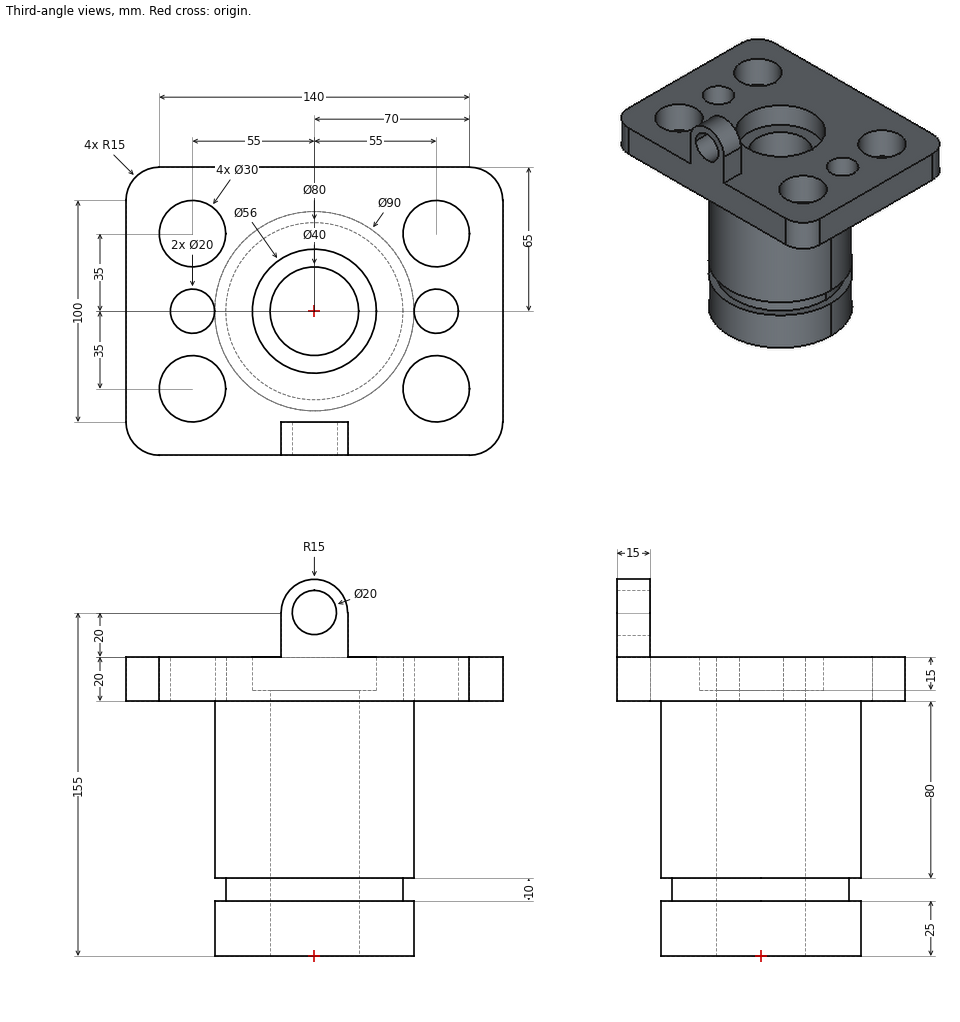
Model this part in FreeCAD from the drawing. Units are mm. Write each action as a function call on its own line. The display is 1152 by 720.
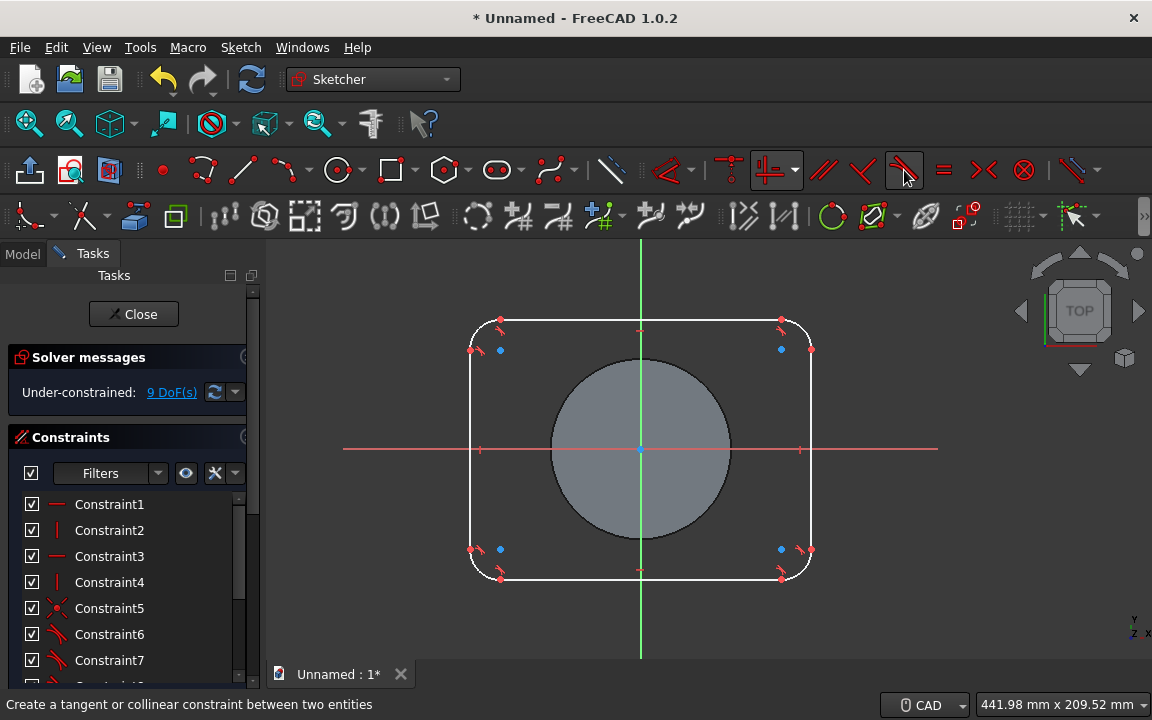
click(811, 490)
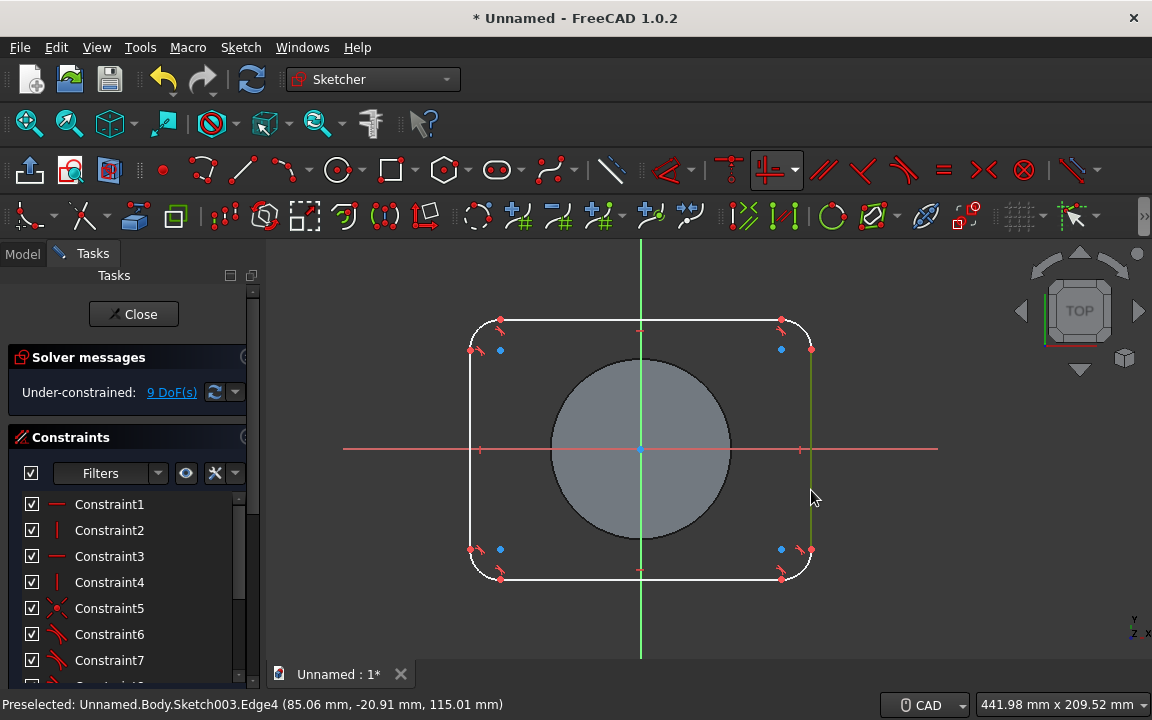
click(808, 336)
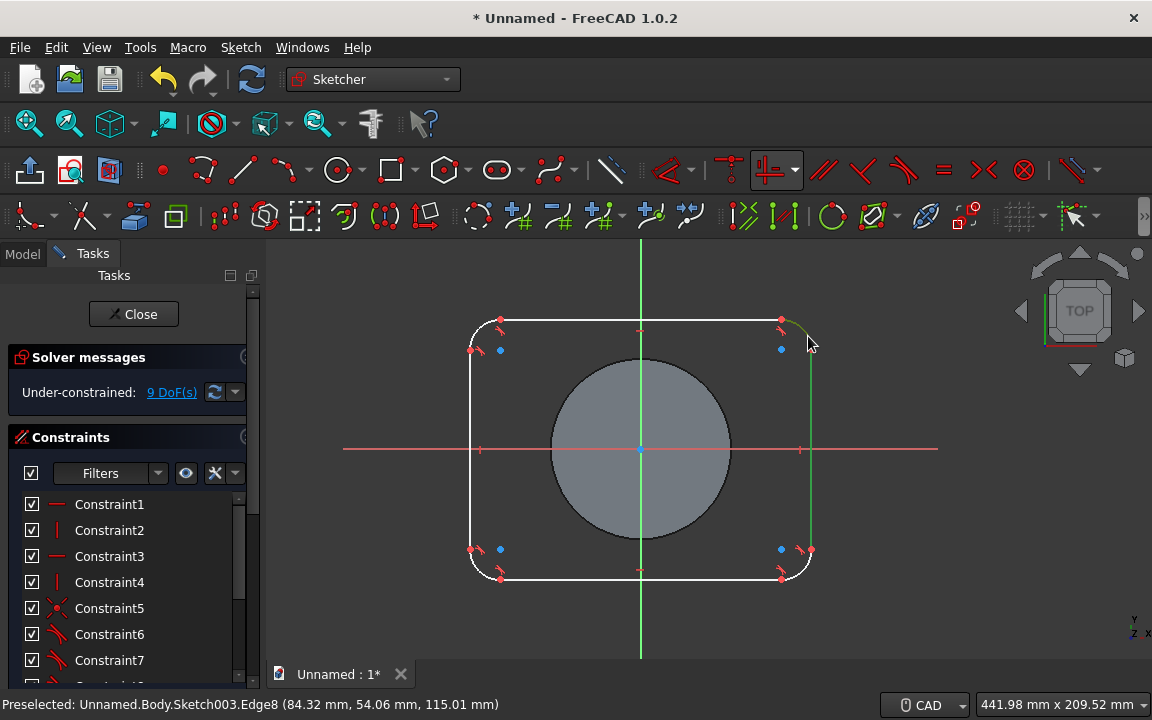
click(904, 170)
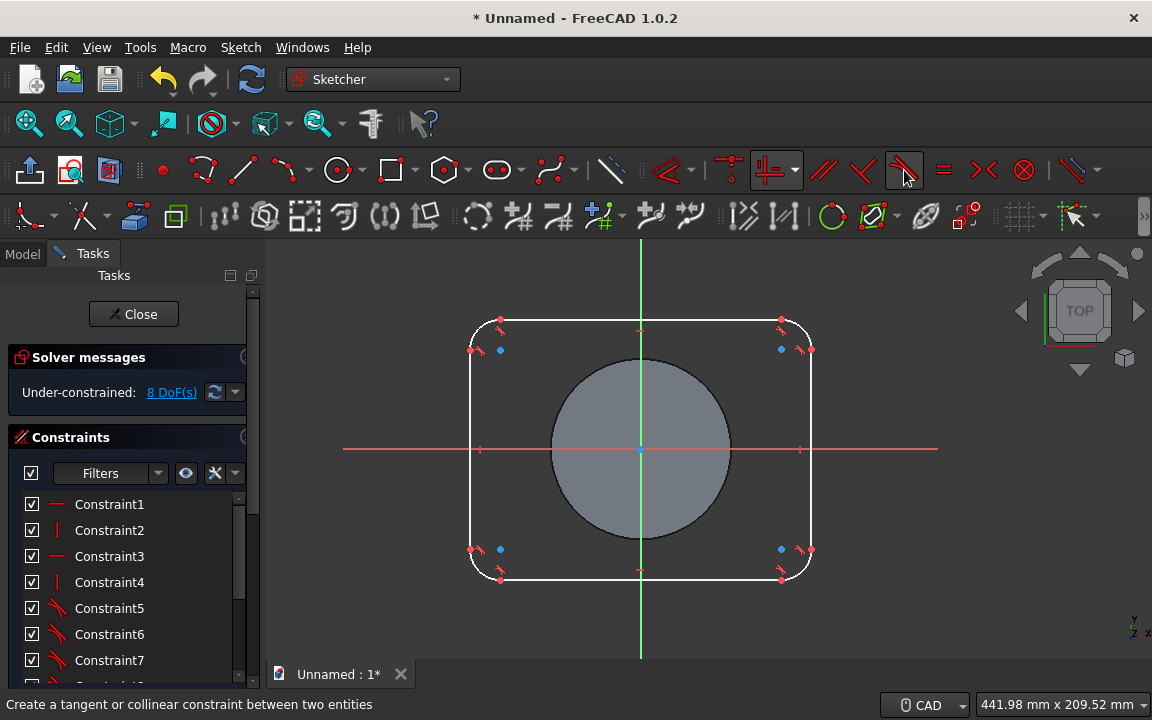
click(487, 323)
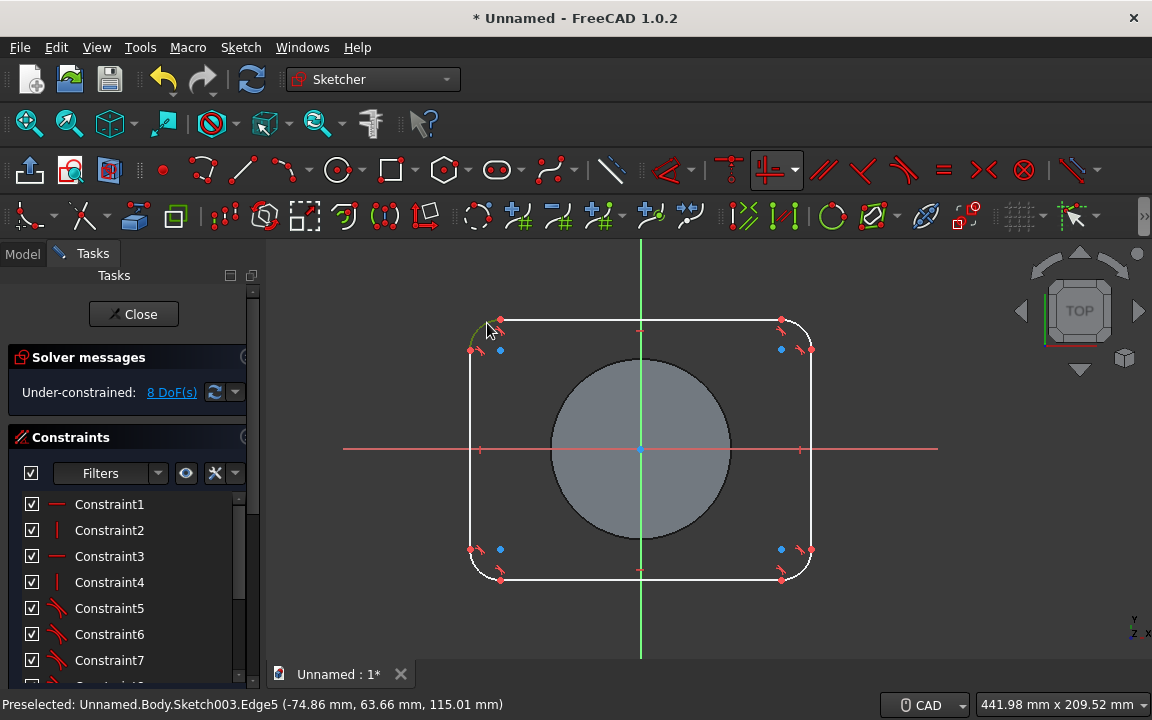
click(473, 563)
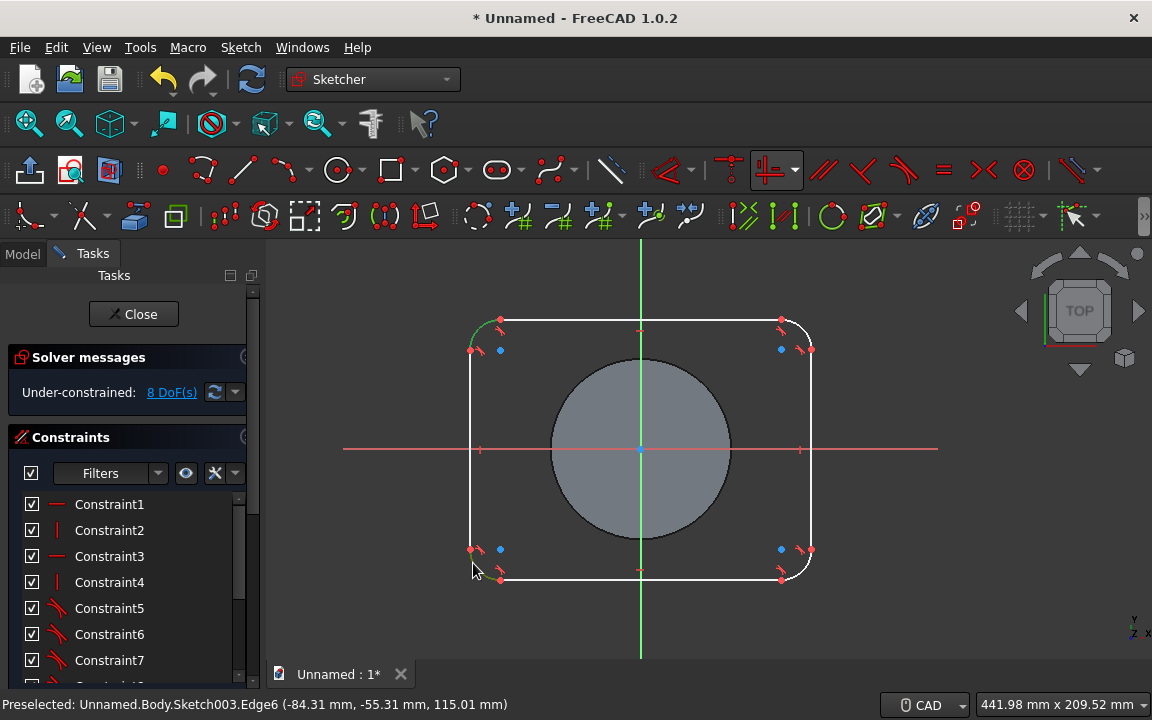
click(795, 577)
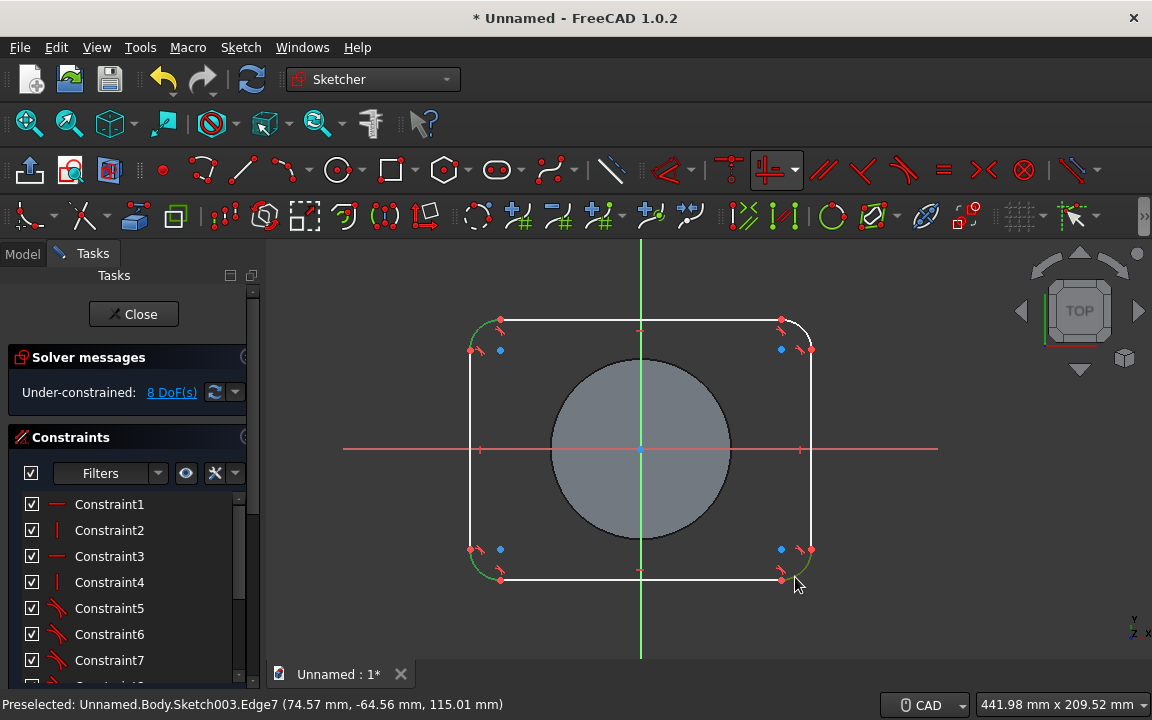
click(808, 336)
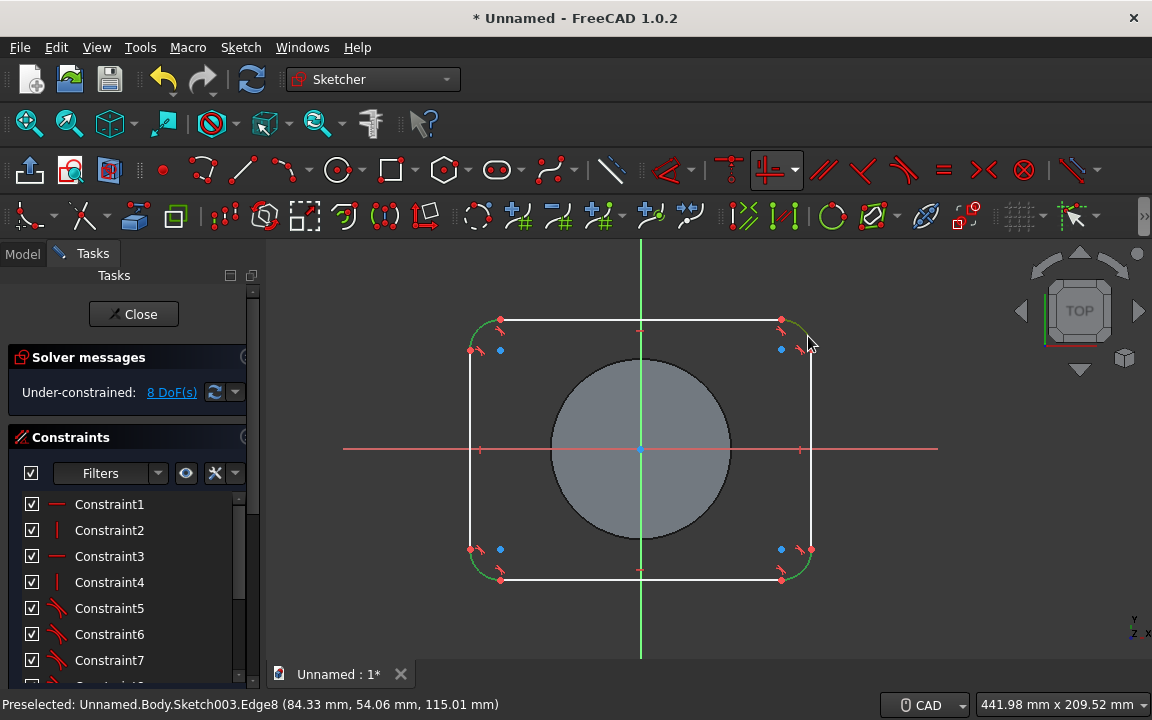
click(944, 170)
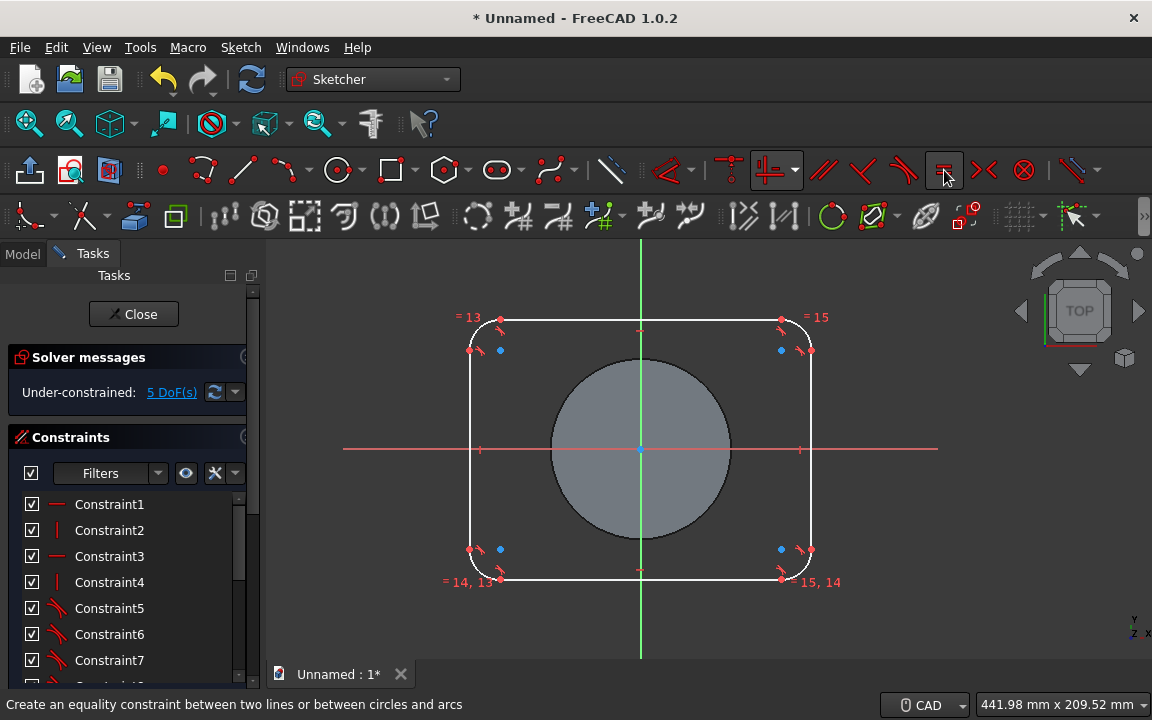
click(666, 170)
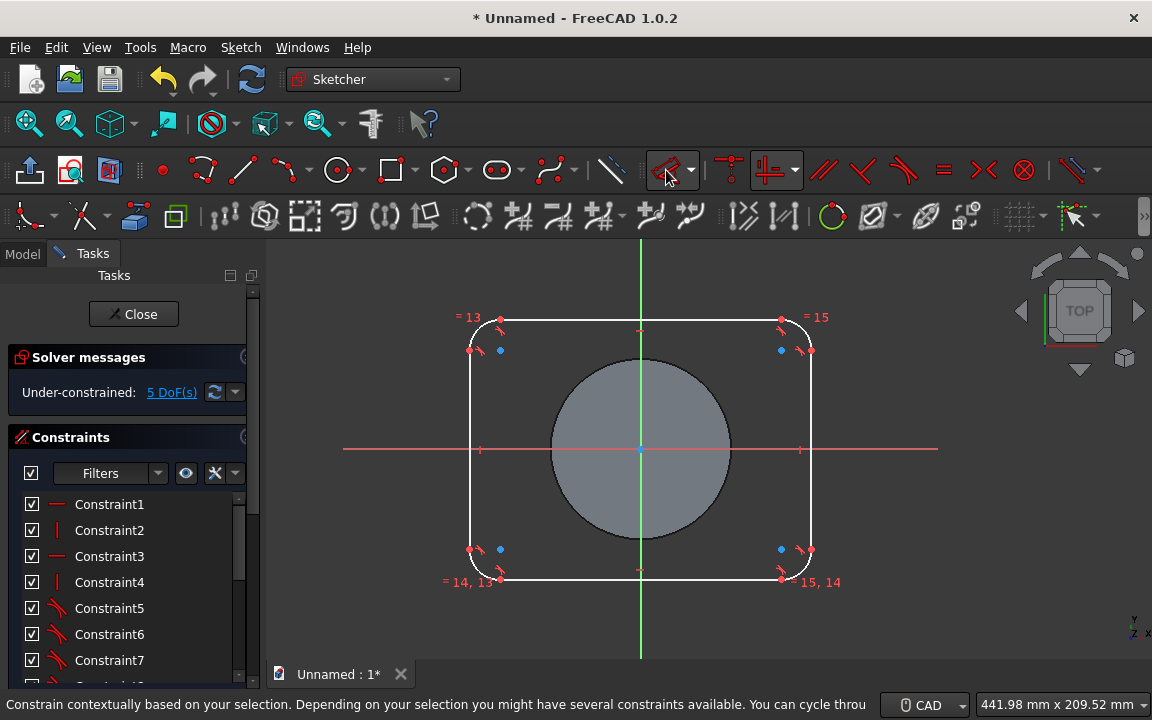
scroll(486, 323, up, 2)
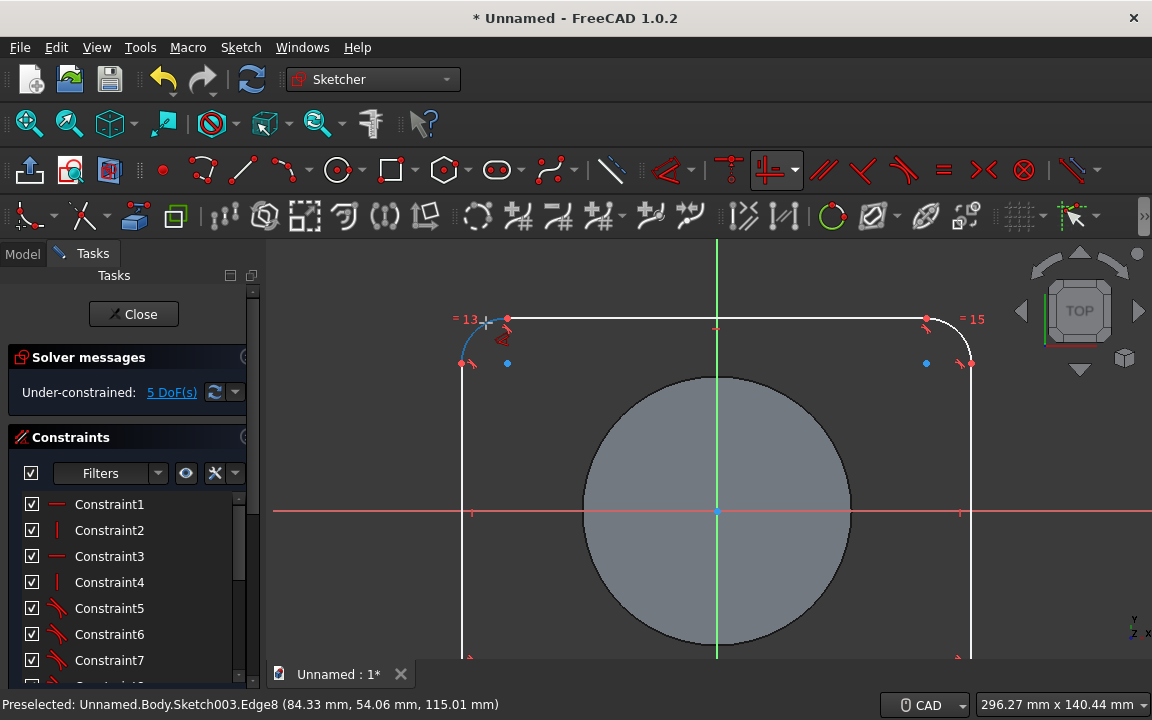
click(486, 323)
click(471, 295)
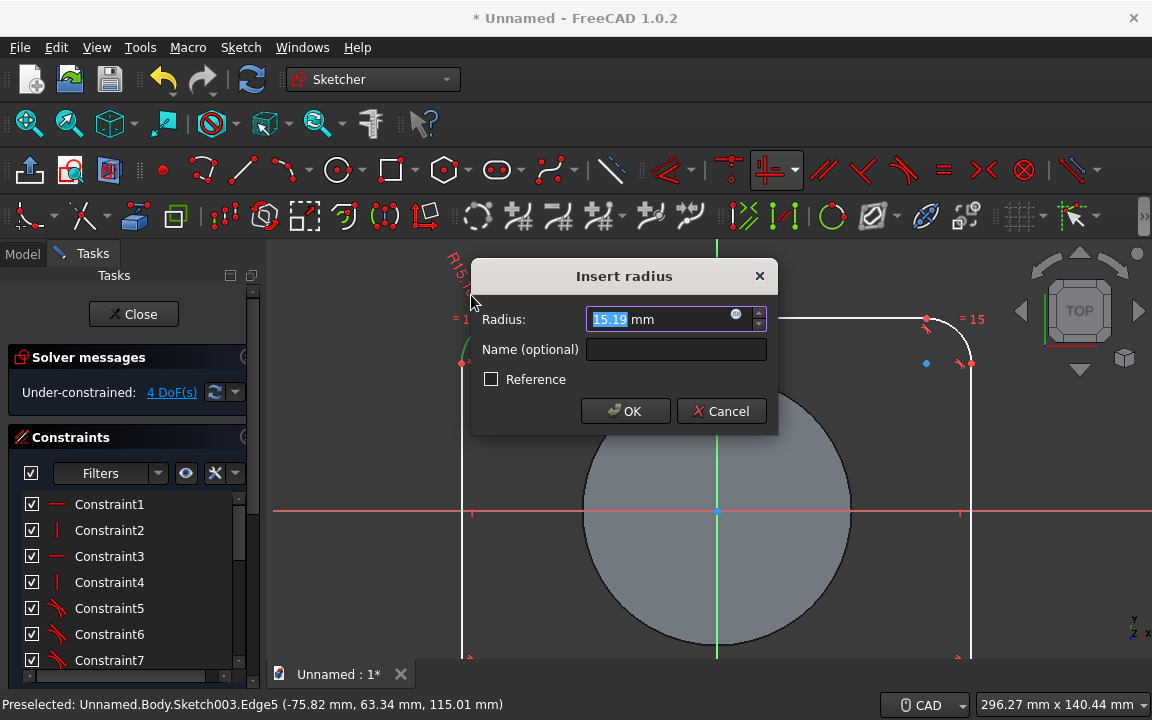
text(15)
key(Return)